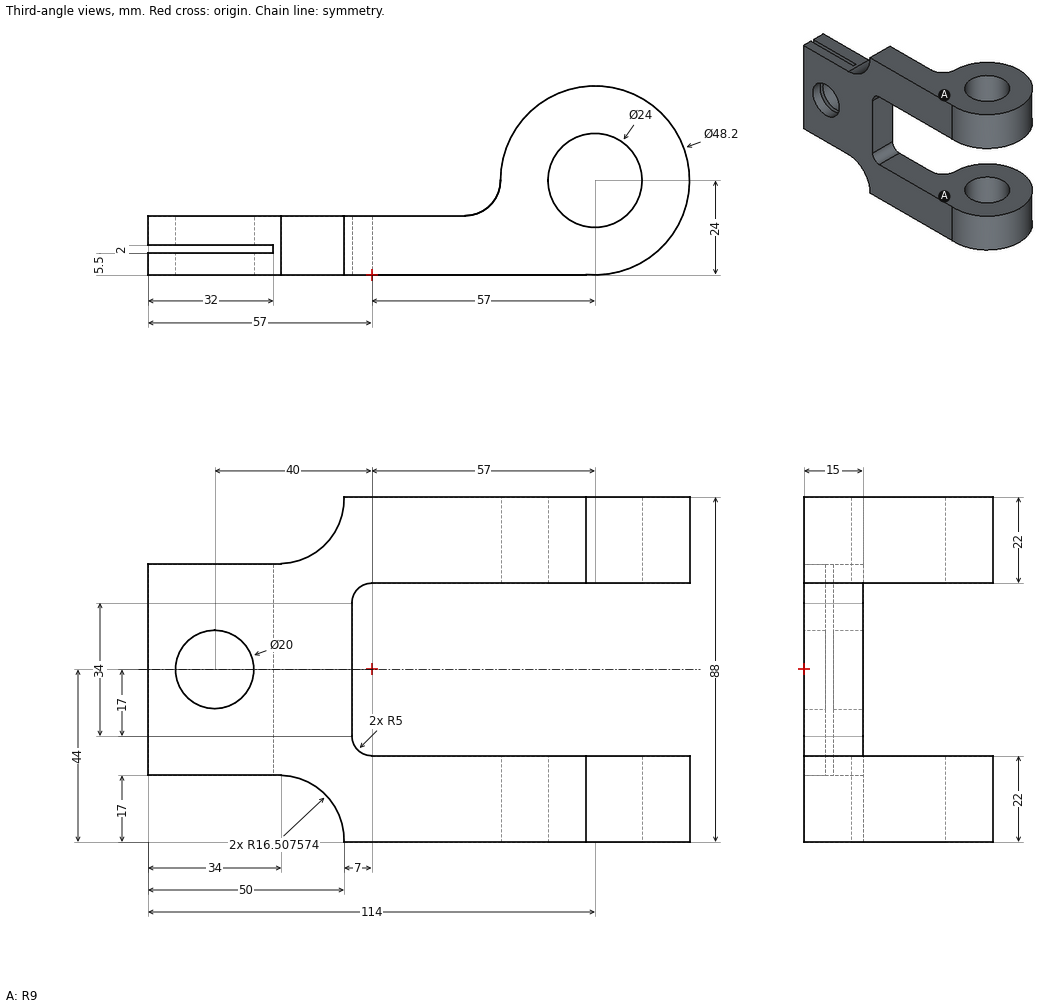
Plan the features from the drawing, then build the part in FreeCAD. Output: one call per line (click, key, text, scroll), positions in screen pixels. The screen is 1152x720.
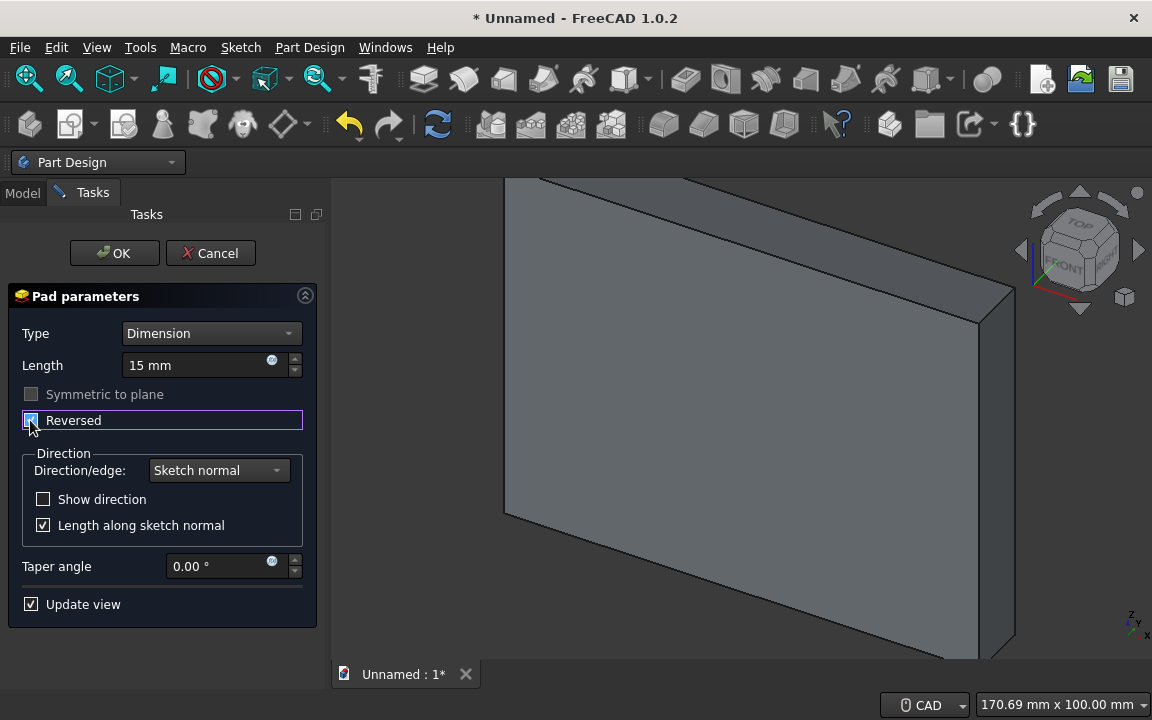
click(115, 253)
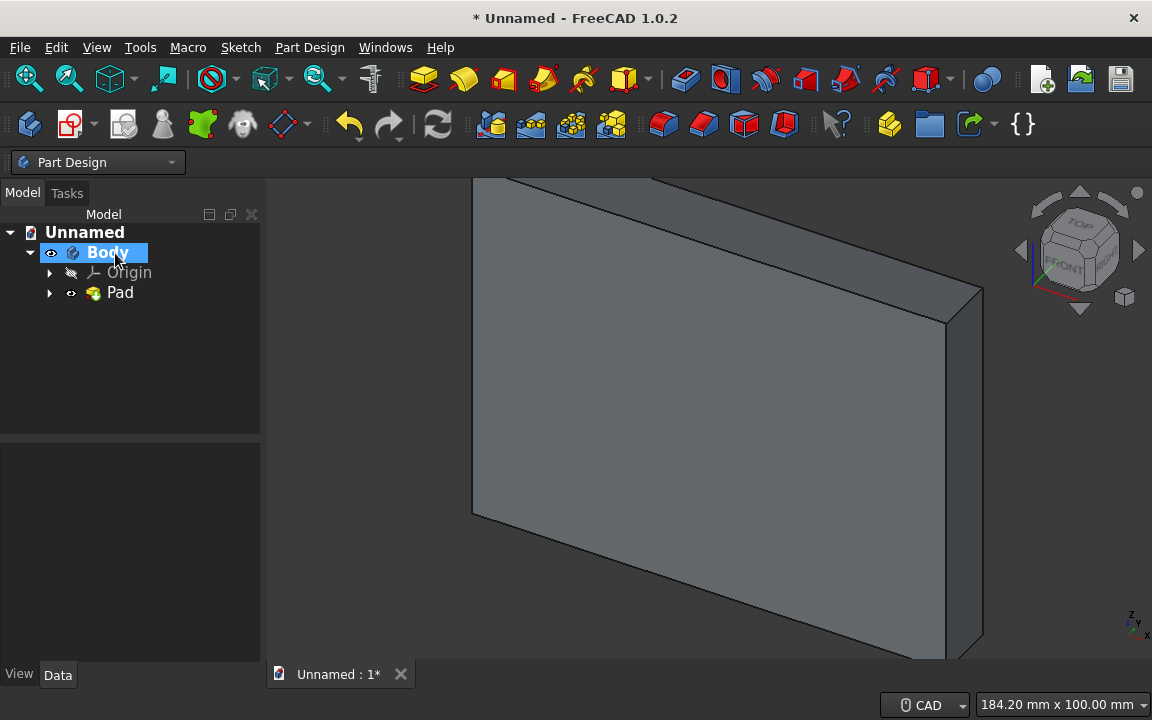
key(v)
key(f)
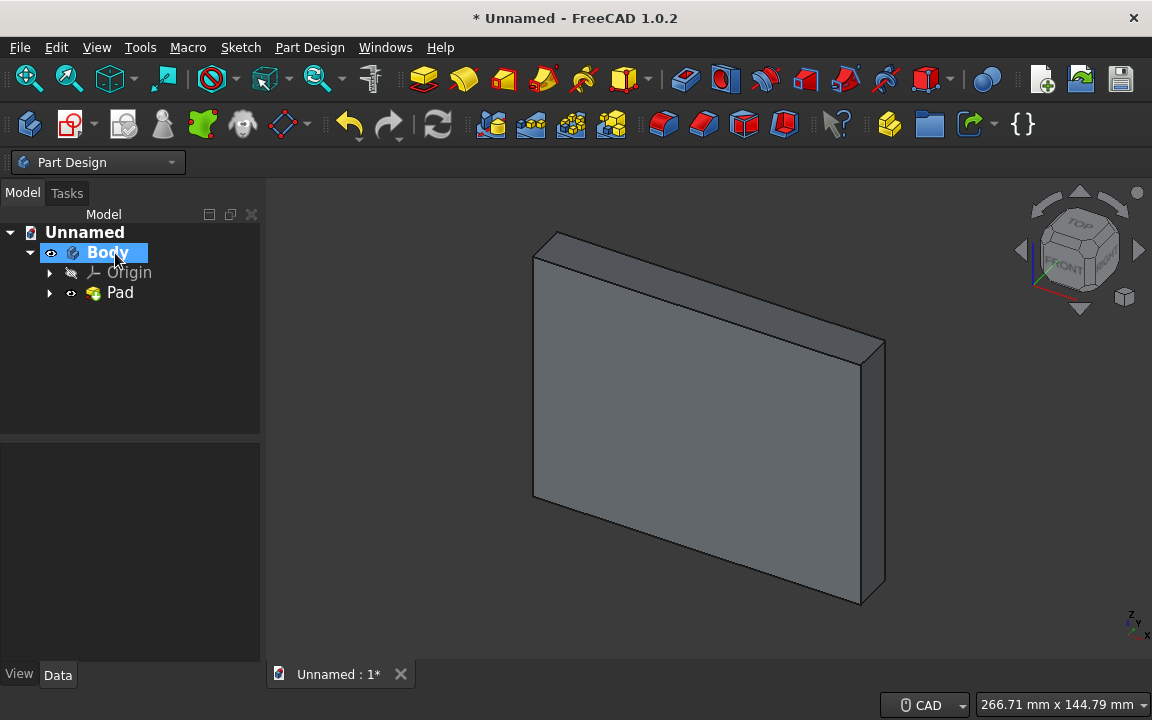
click(850, 344)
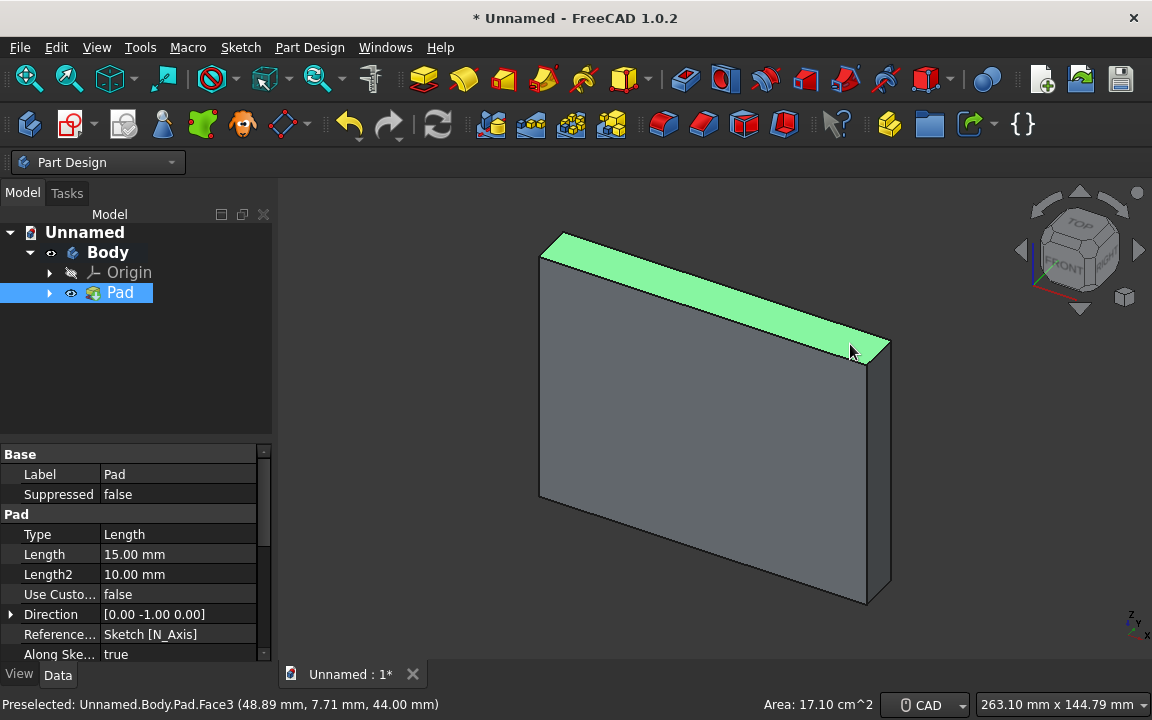
click(70, 124)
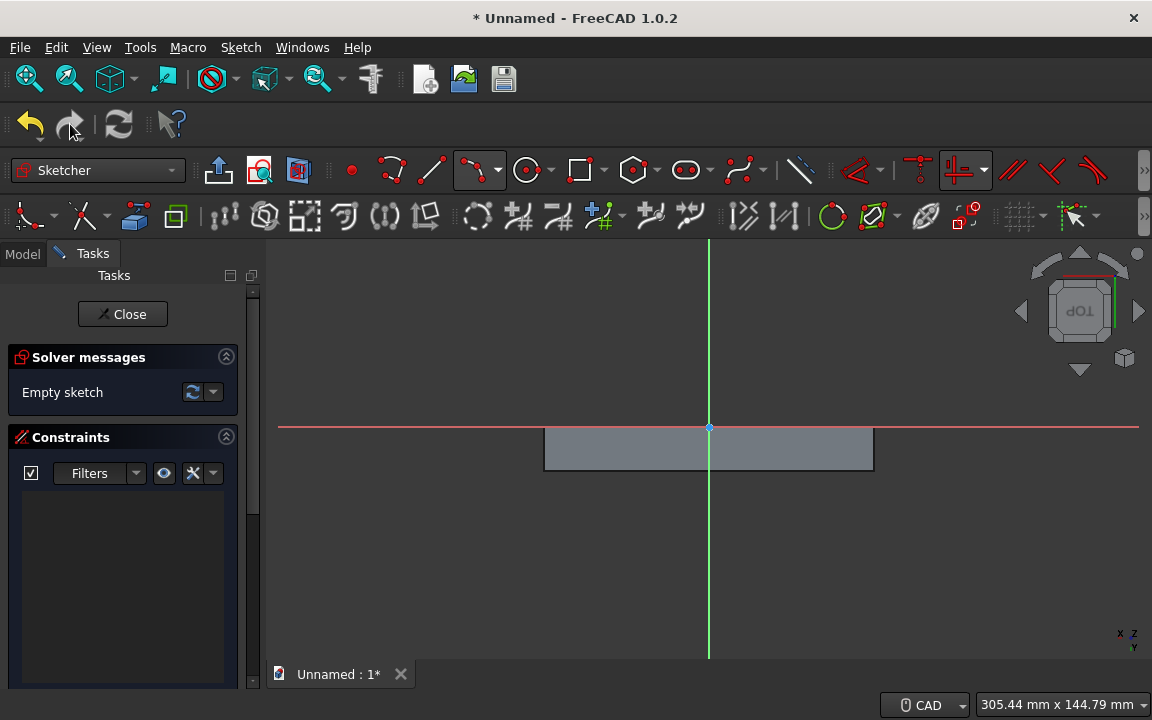
scroll(532, 555, up, 3)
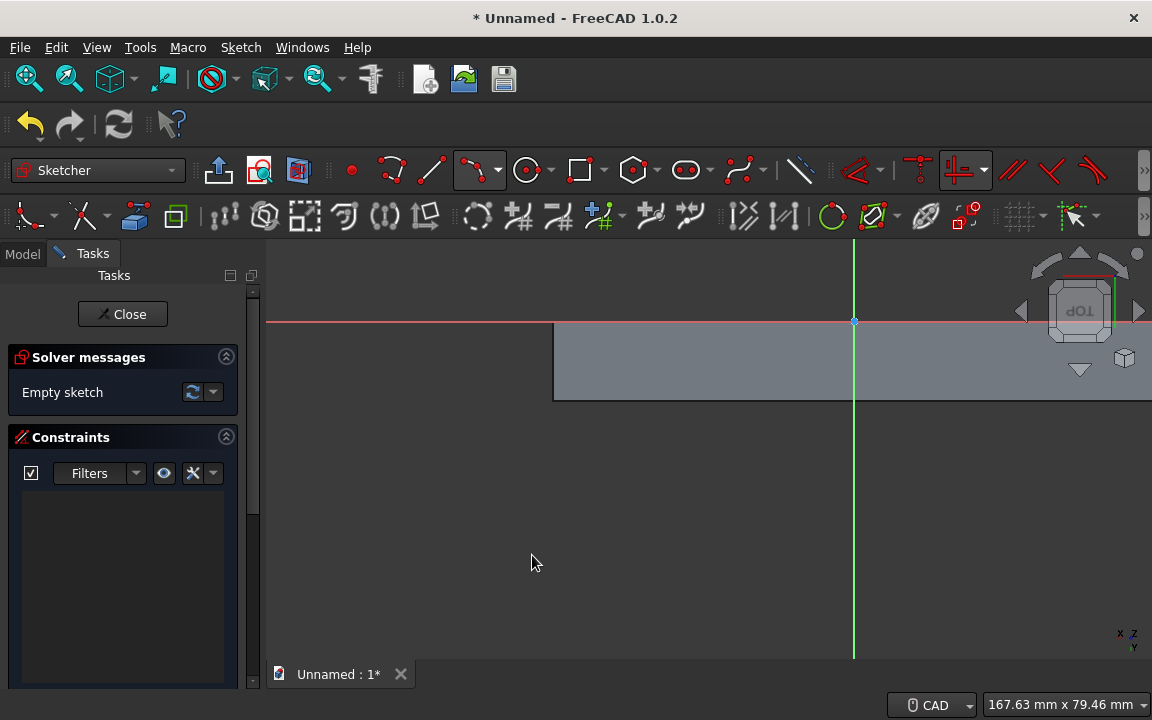
key(g)
key(c)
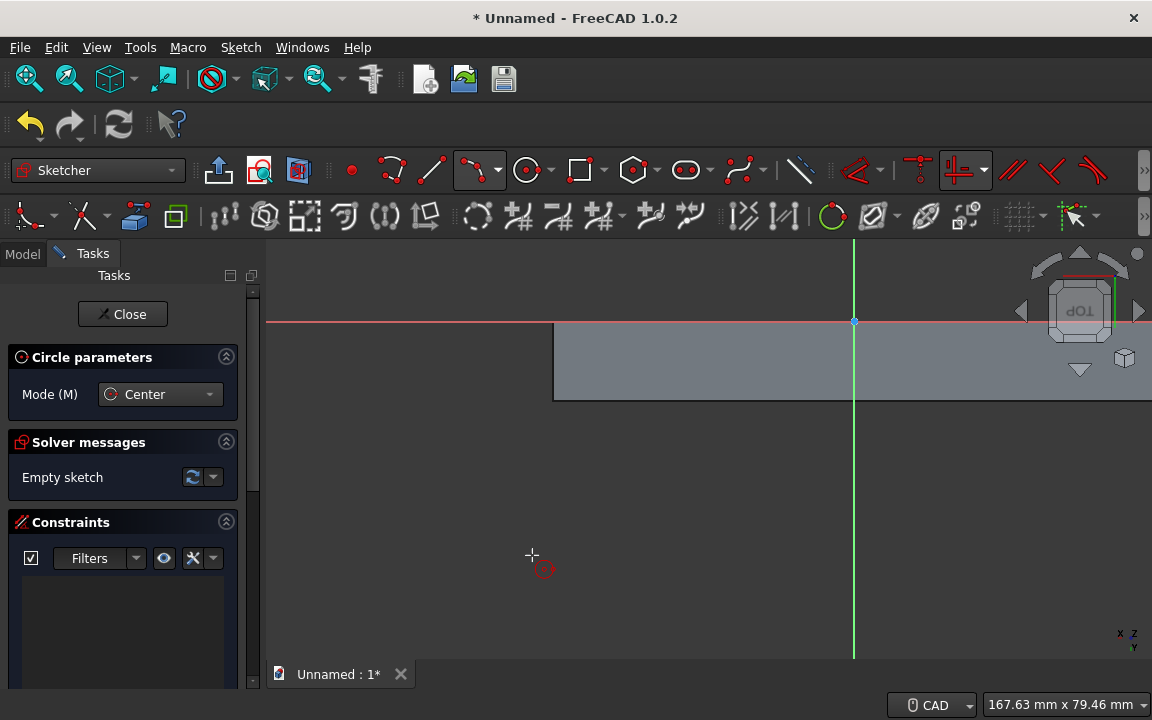
click(553, 448)
move(643, 358)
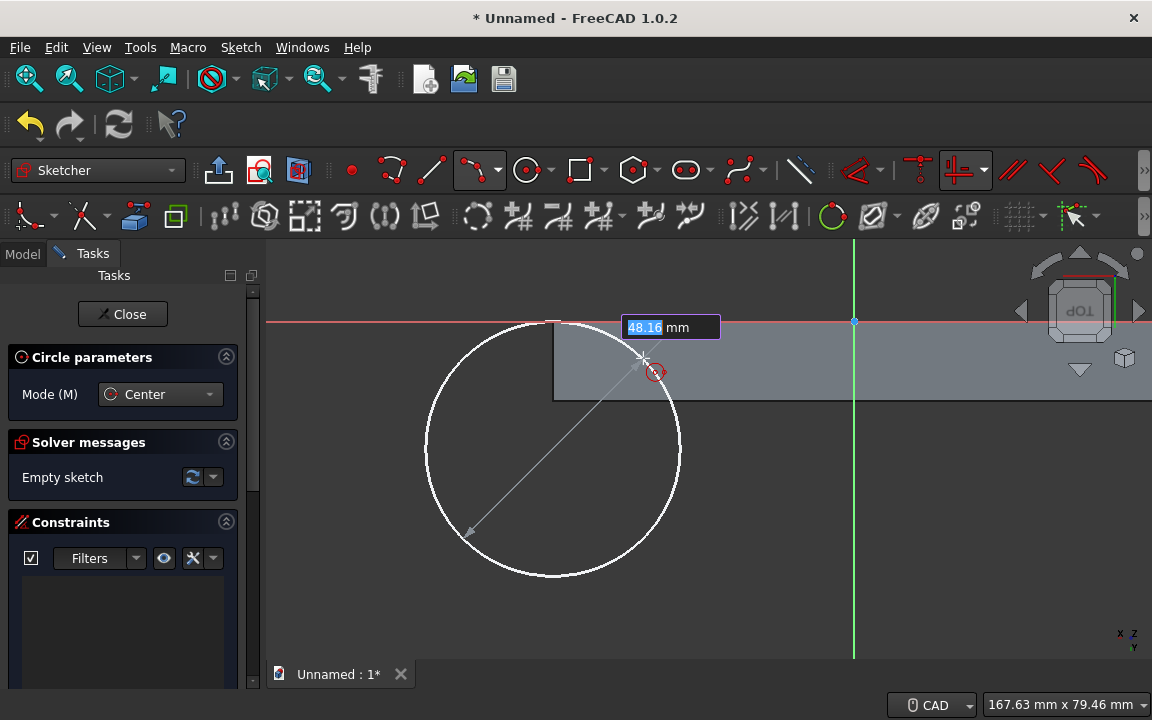
text(48.2)
key(Return)
key(Escape)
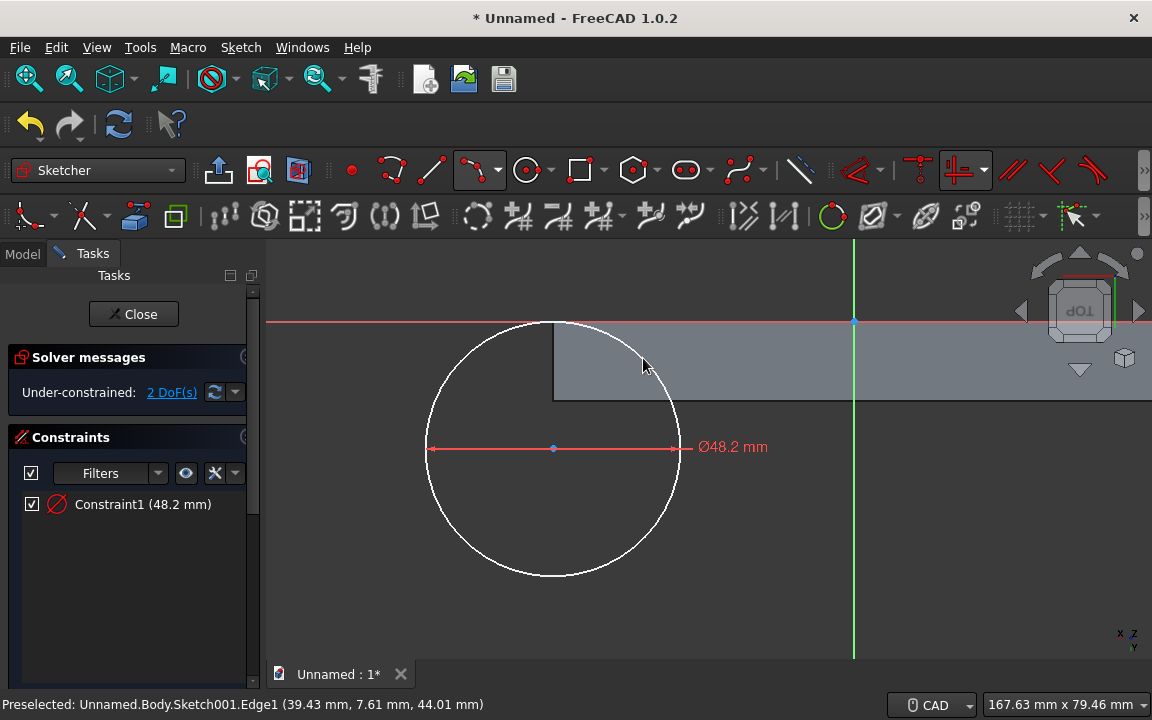
key(d)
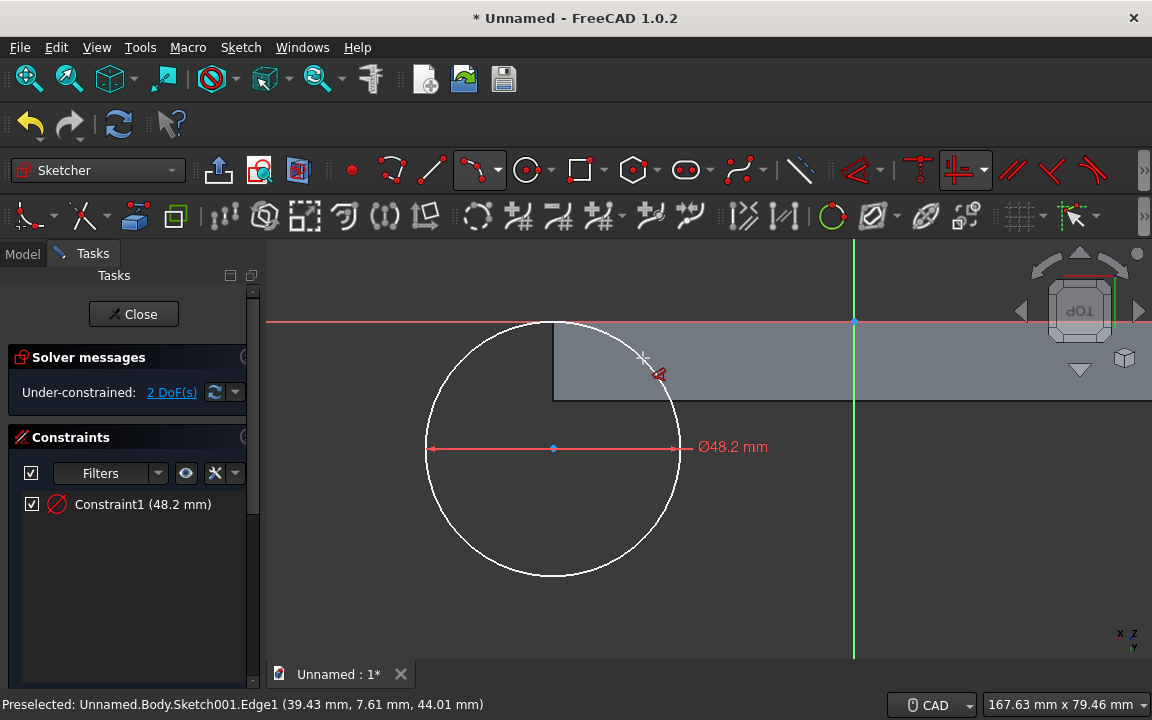
click(553, 449)
click(704, 288)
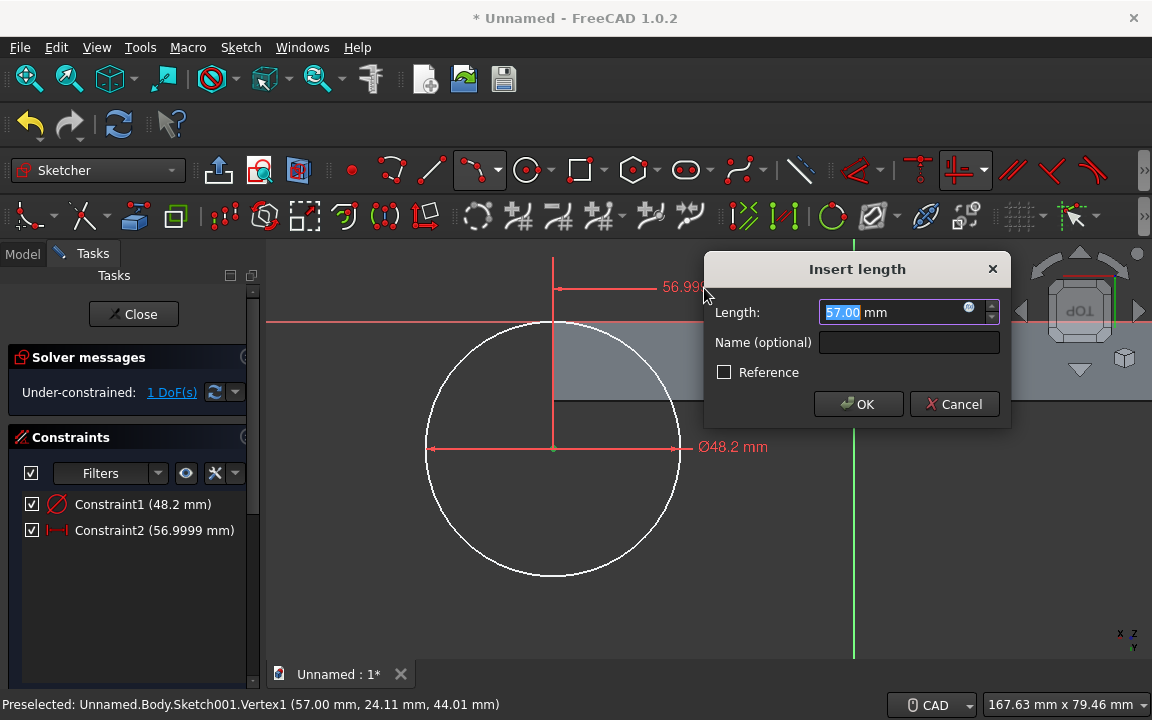
text(57)
key(Return)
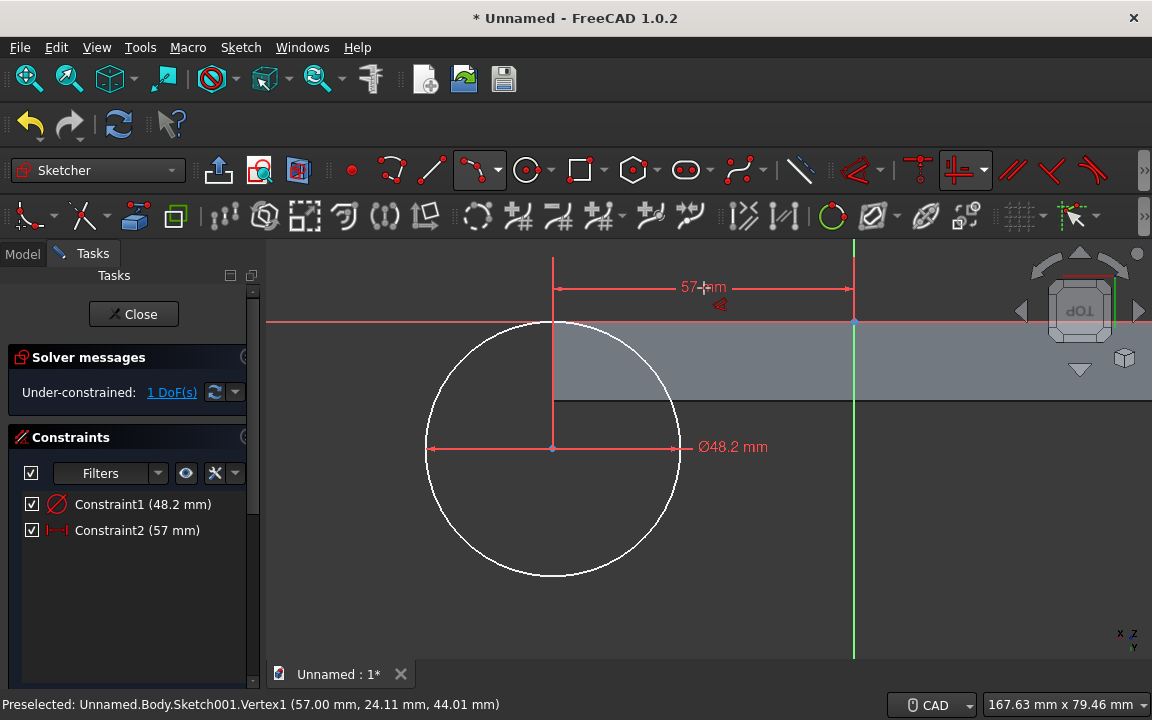
click(553, 449)
click(888, 385)